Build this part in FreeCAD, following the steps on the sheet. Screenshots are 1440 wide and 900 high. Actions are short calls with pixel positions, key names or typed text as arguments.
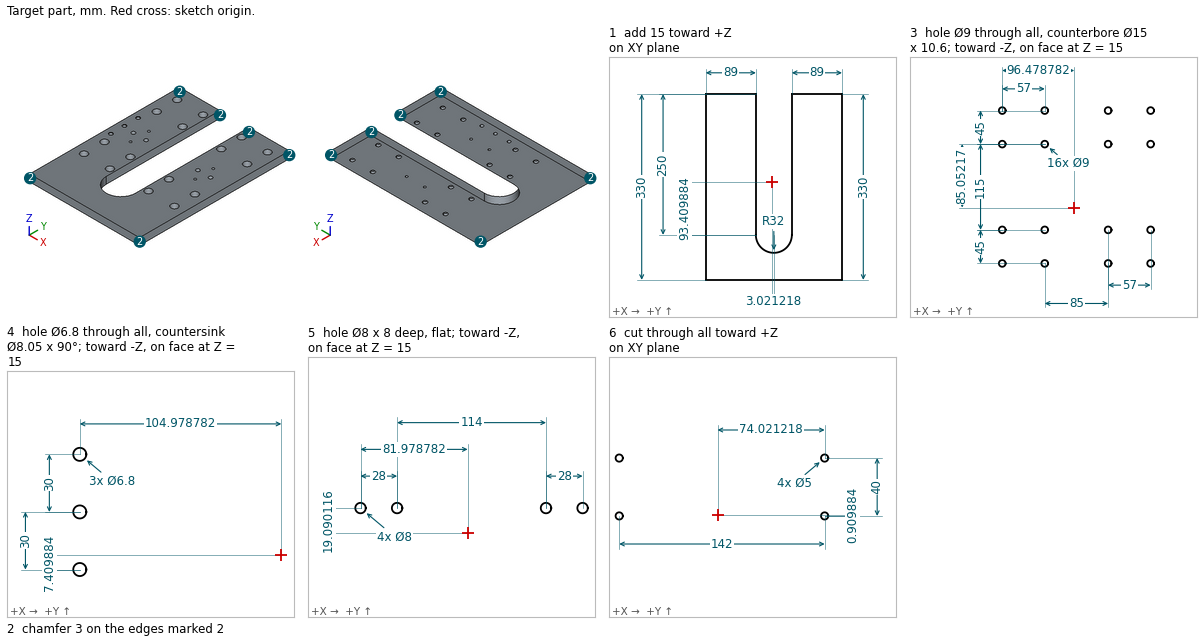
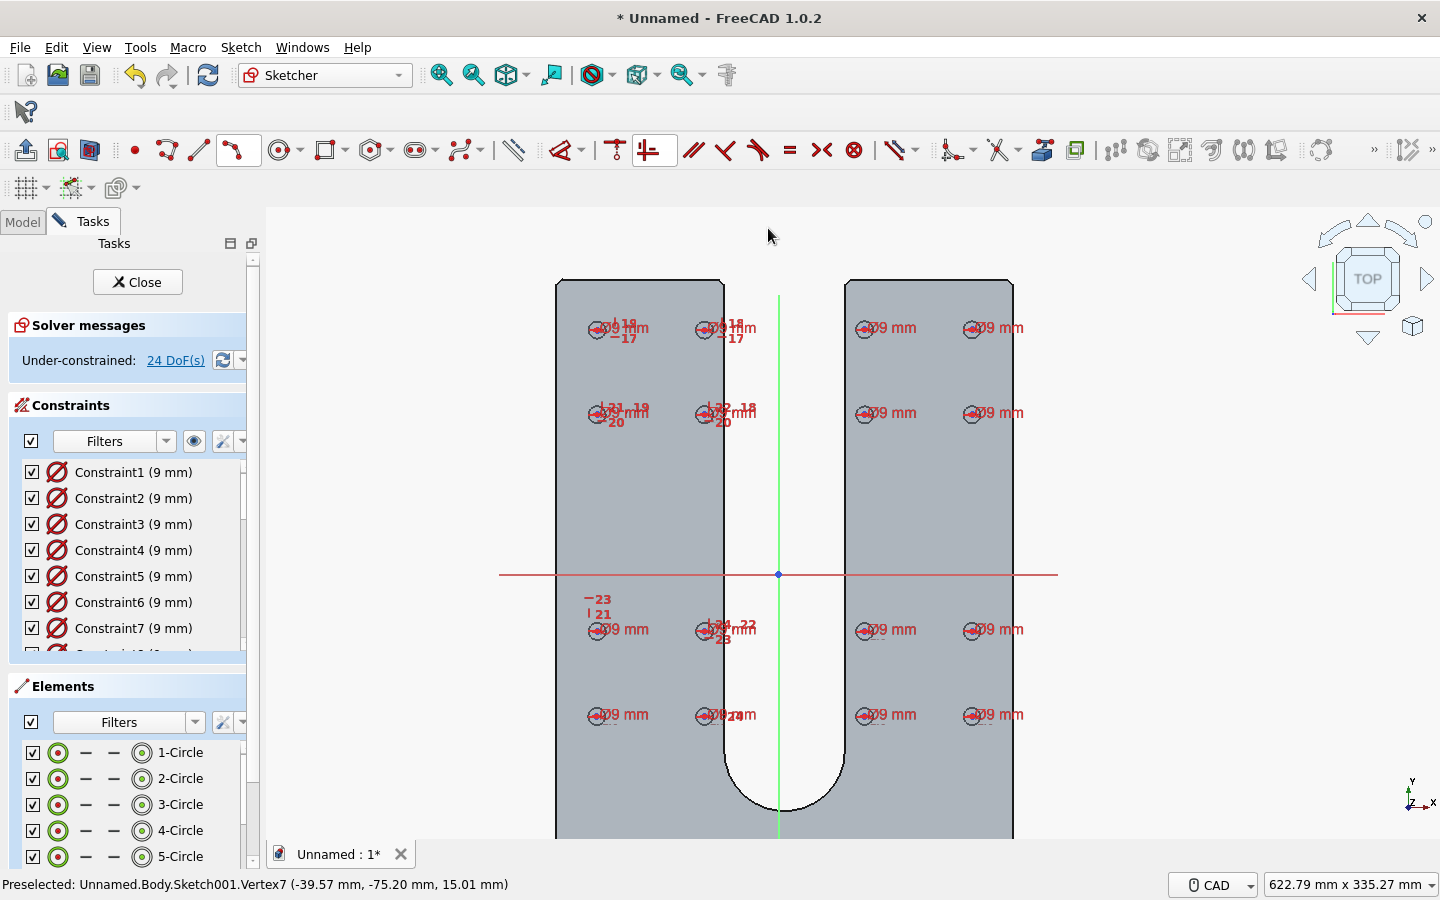
click(597, 631)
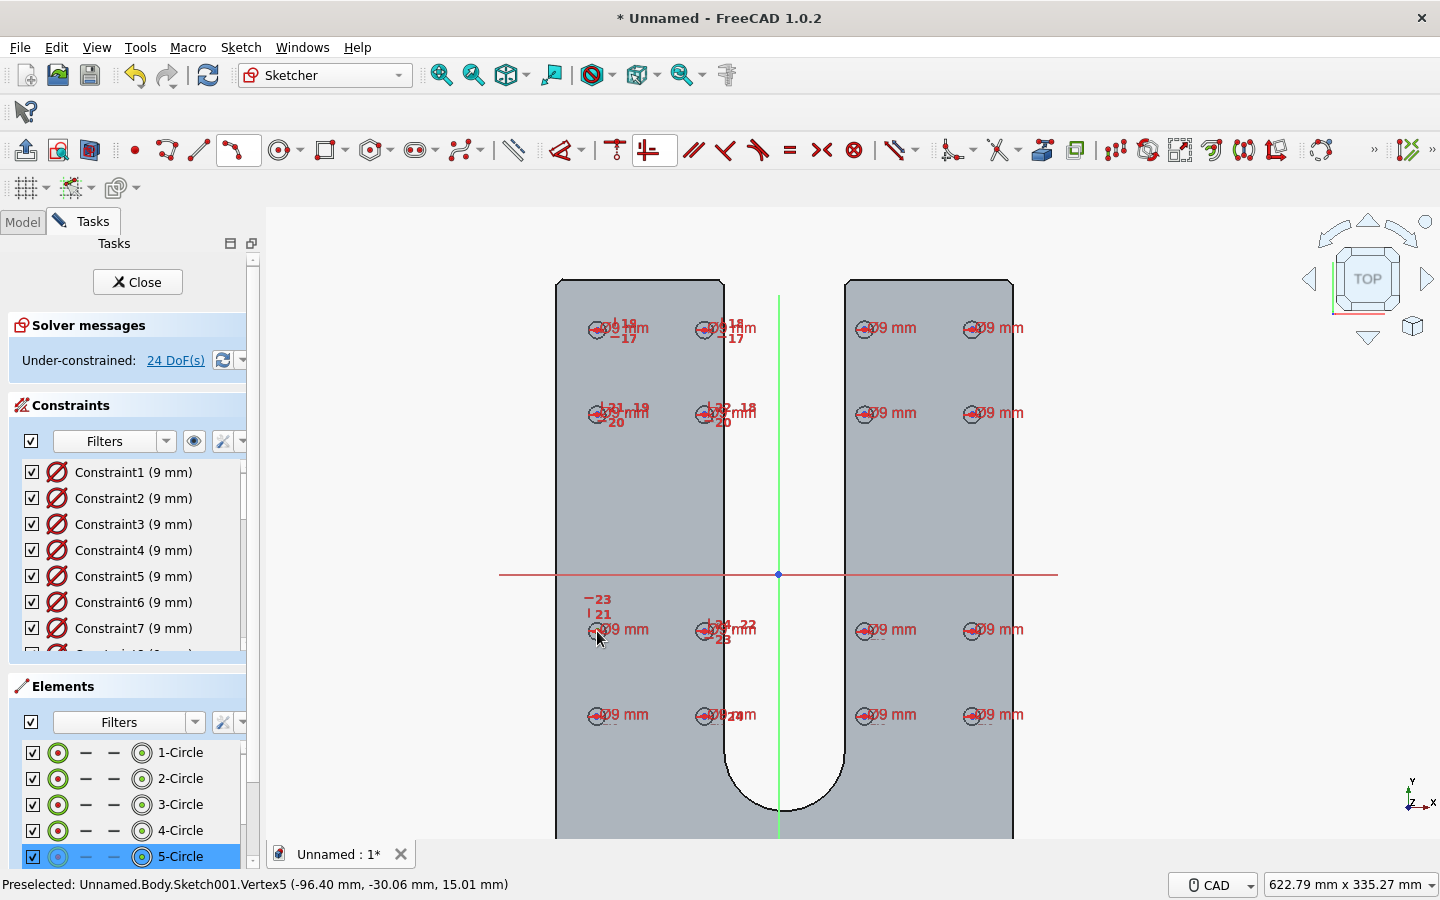
click(597, 717)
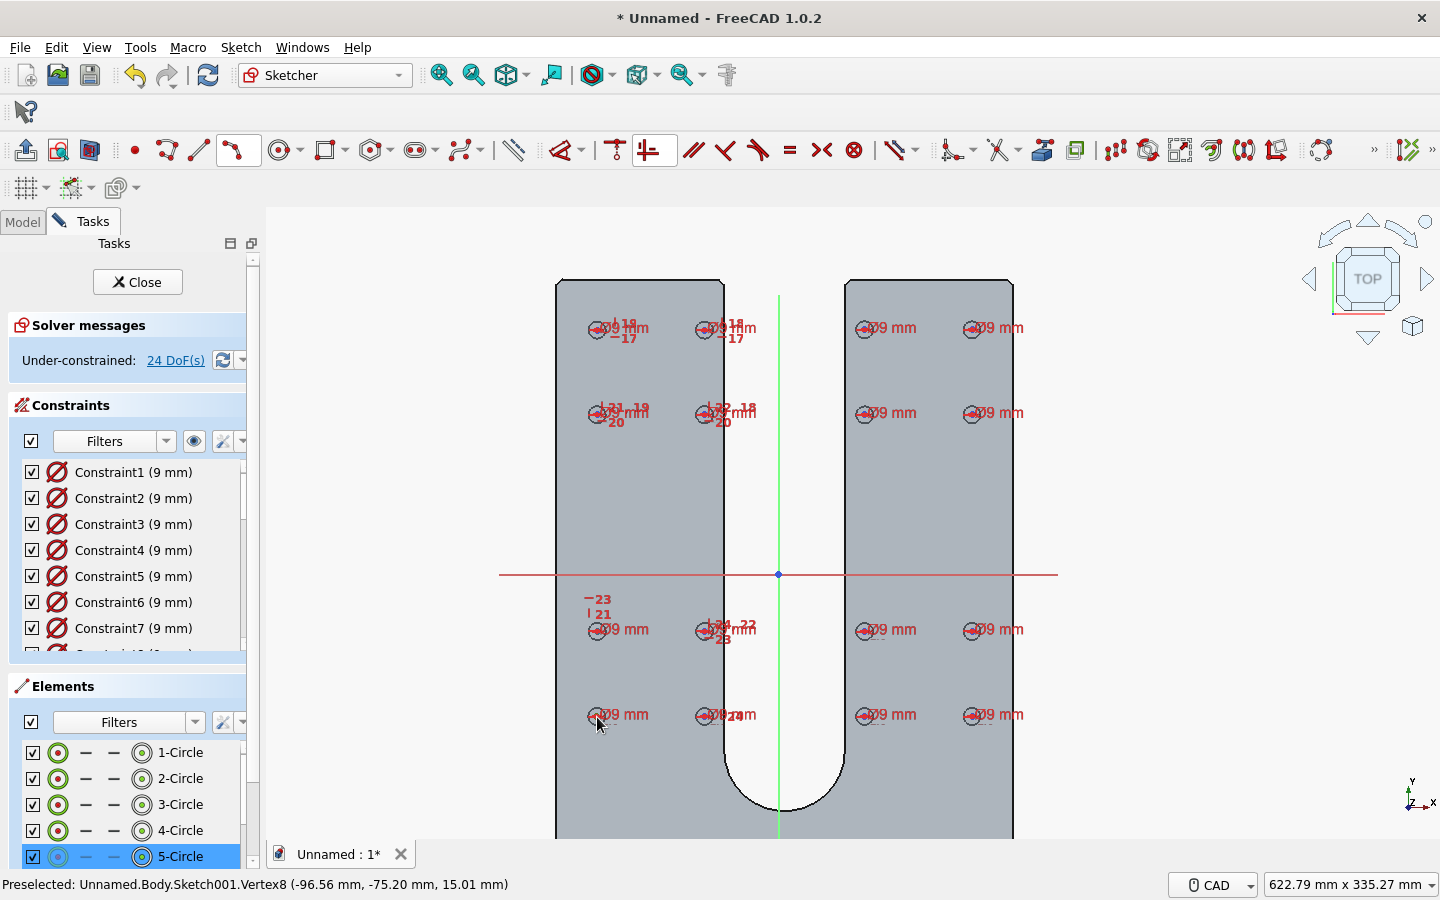
click(672, 150)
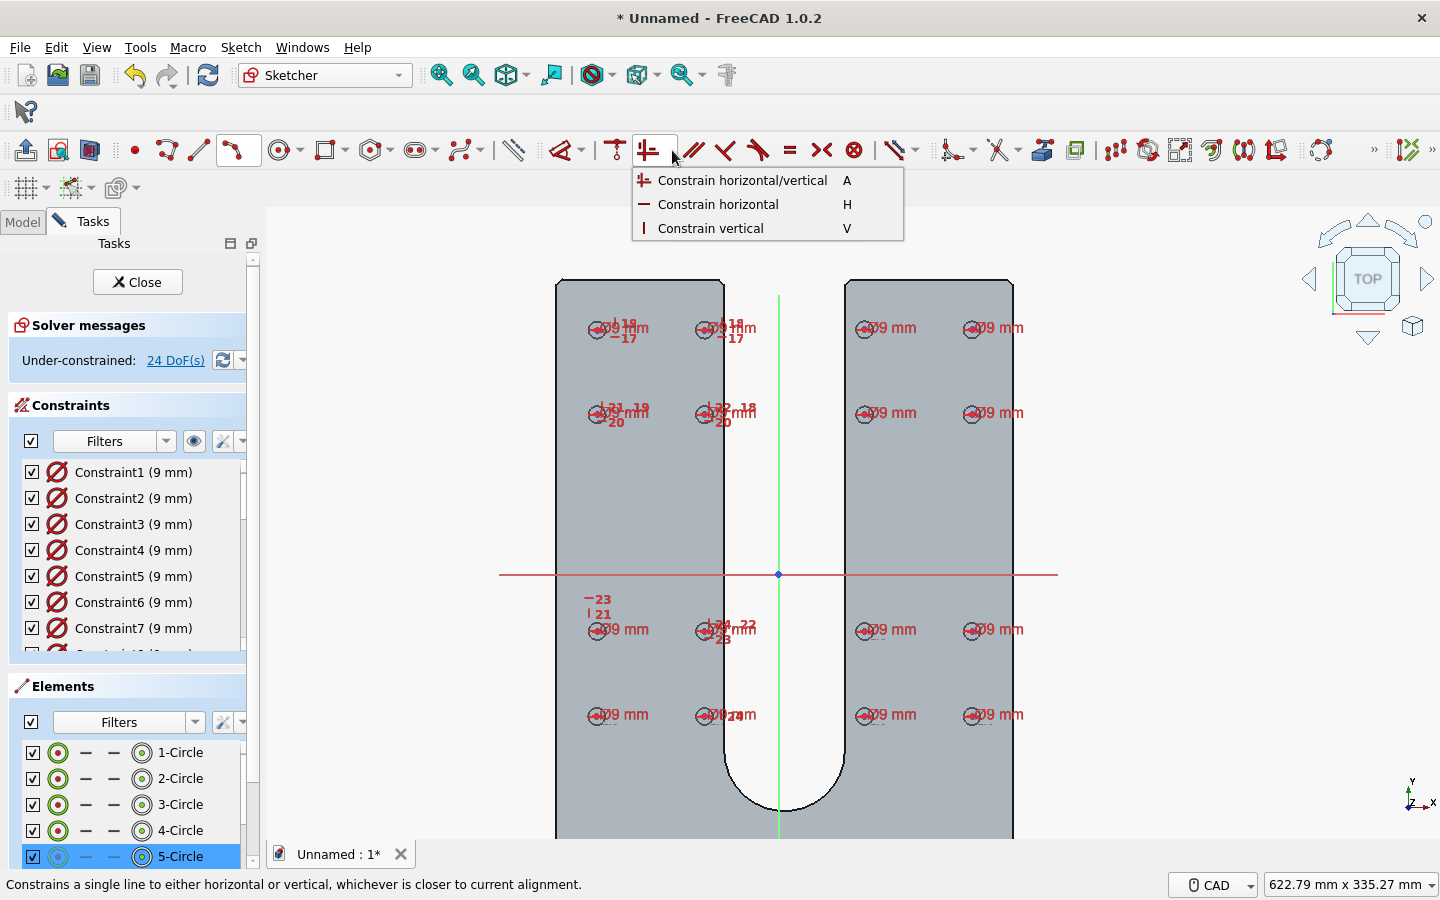
click(768, 228)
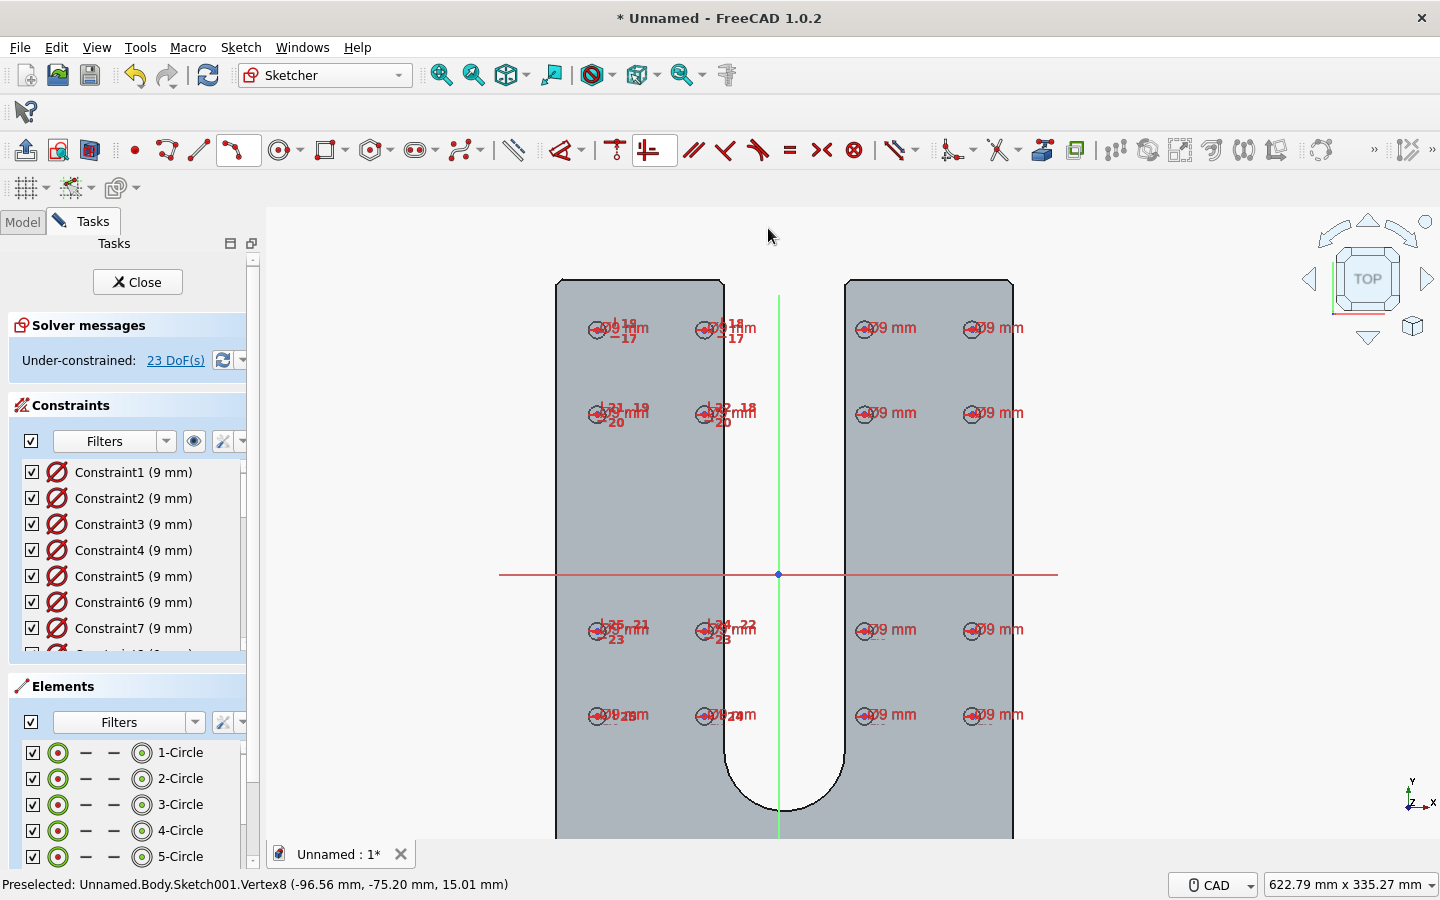
click(705, 717)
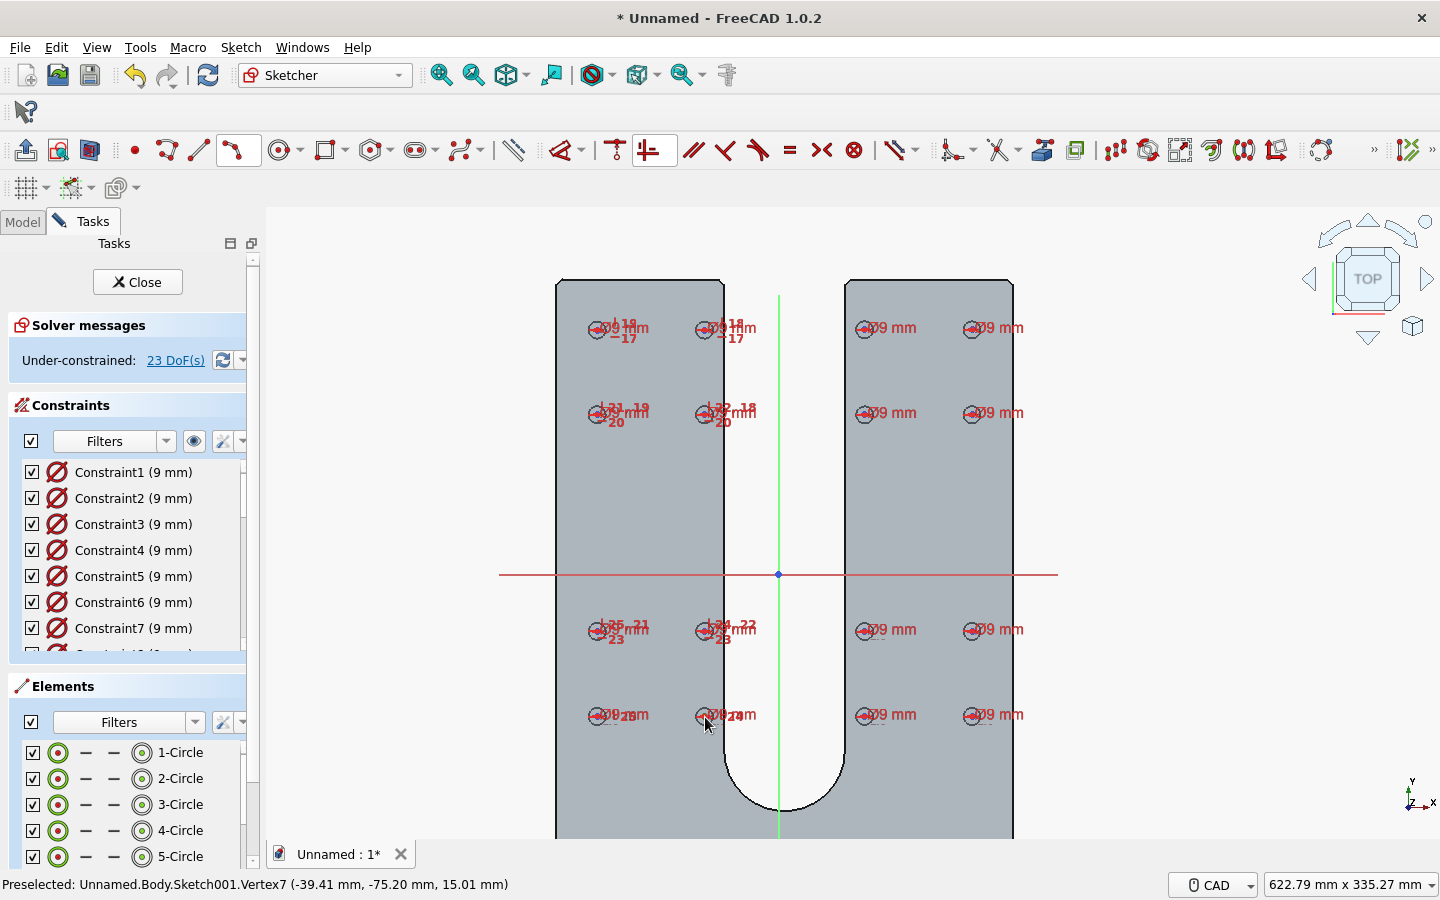
click(597, 717)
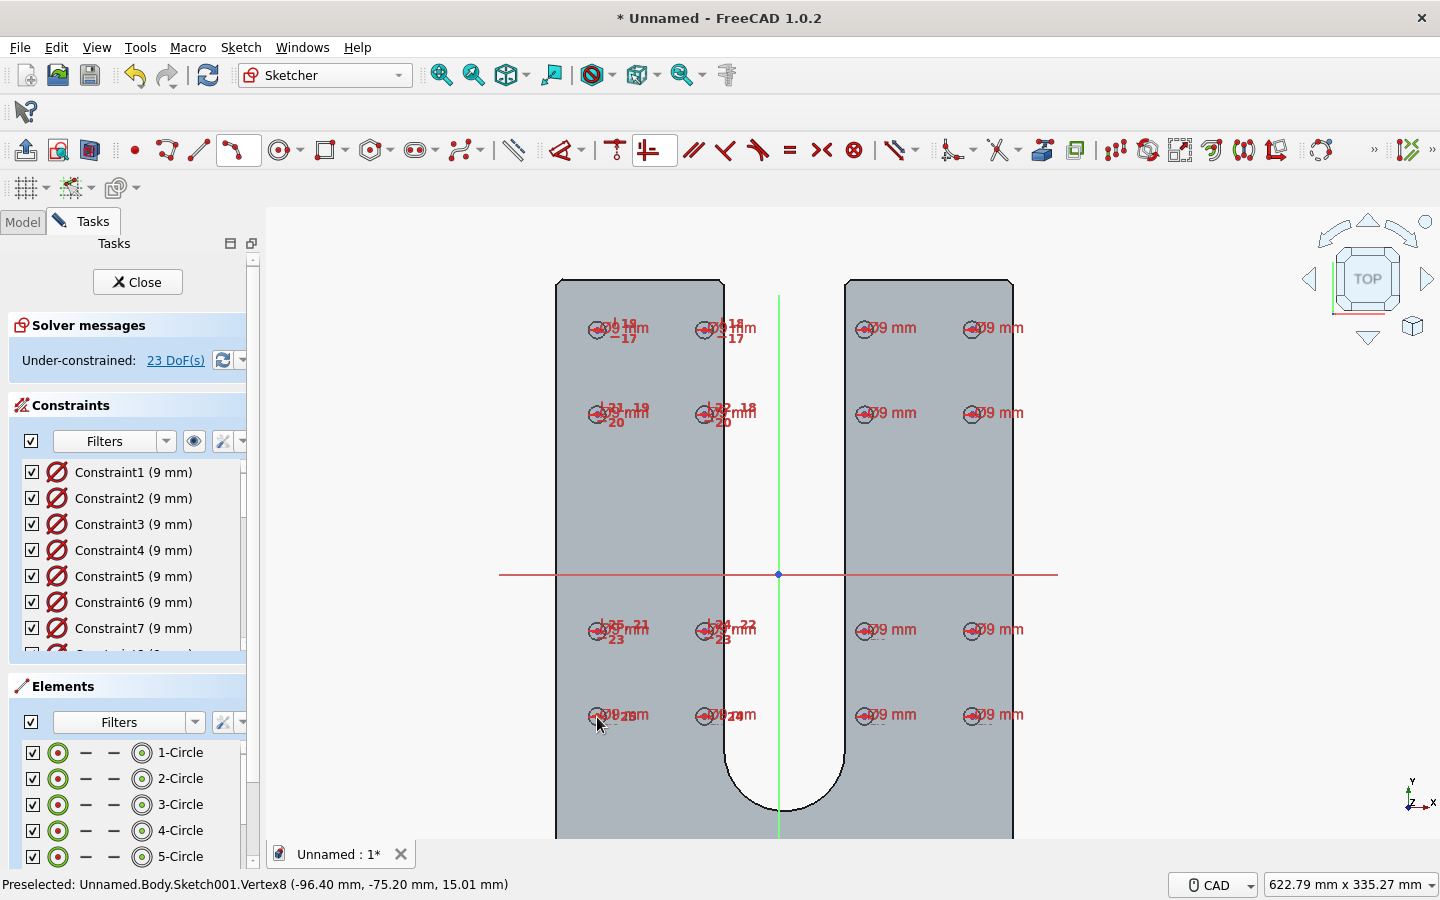
click(672, 150)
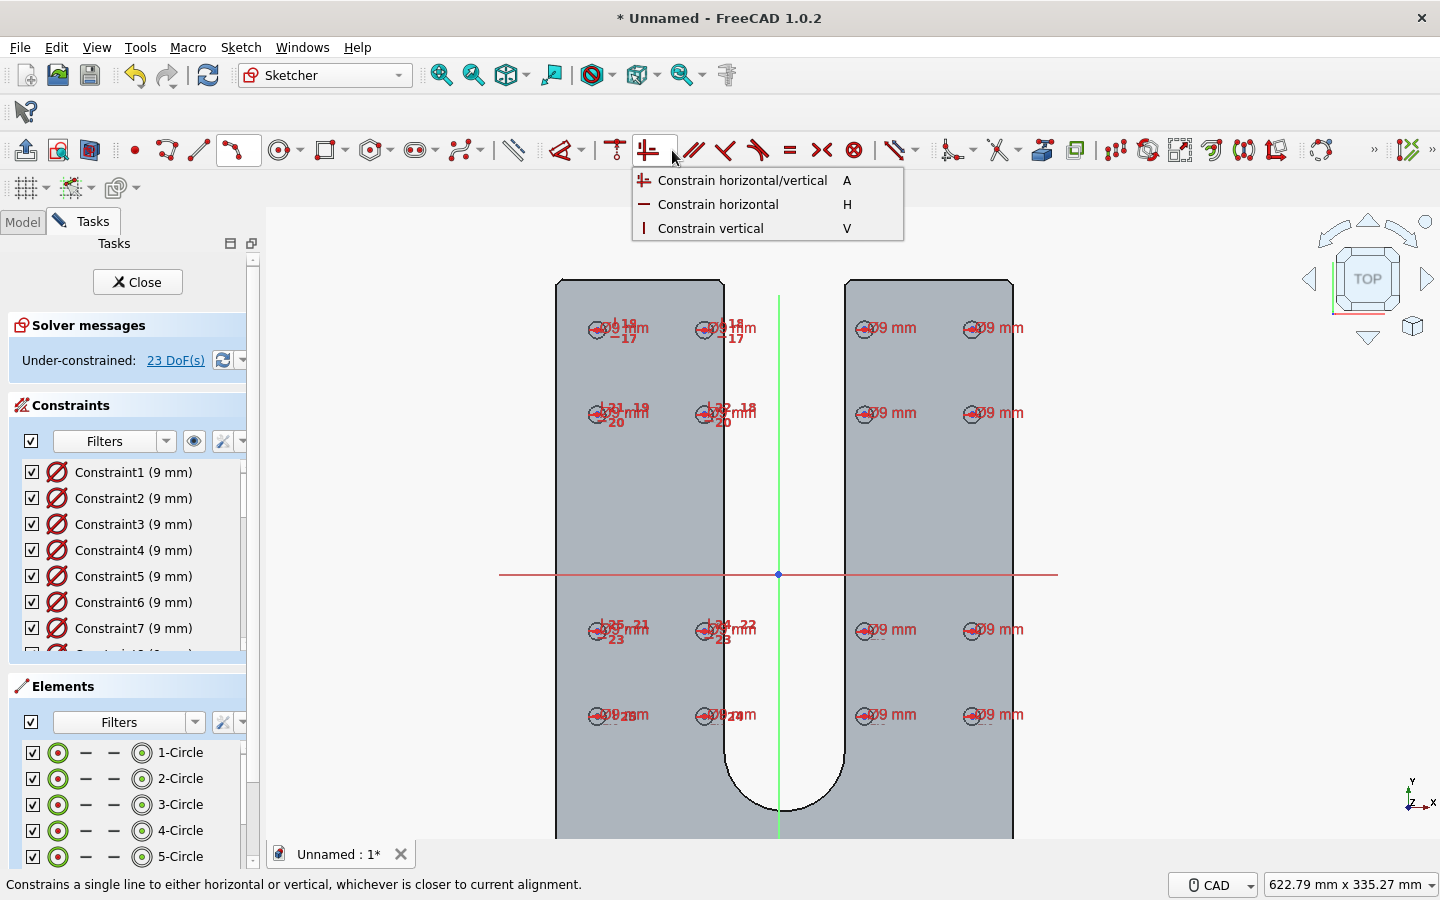
click(768, 204)